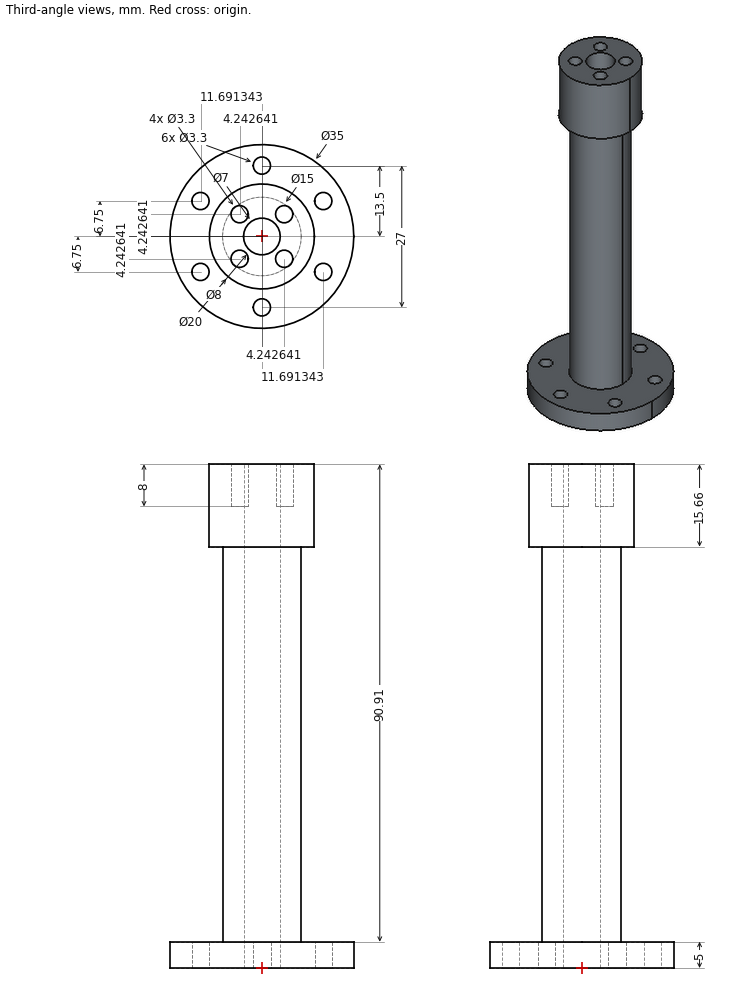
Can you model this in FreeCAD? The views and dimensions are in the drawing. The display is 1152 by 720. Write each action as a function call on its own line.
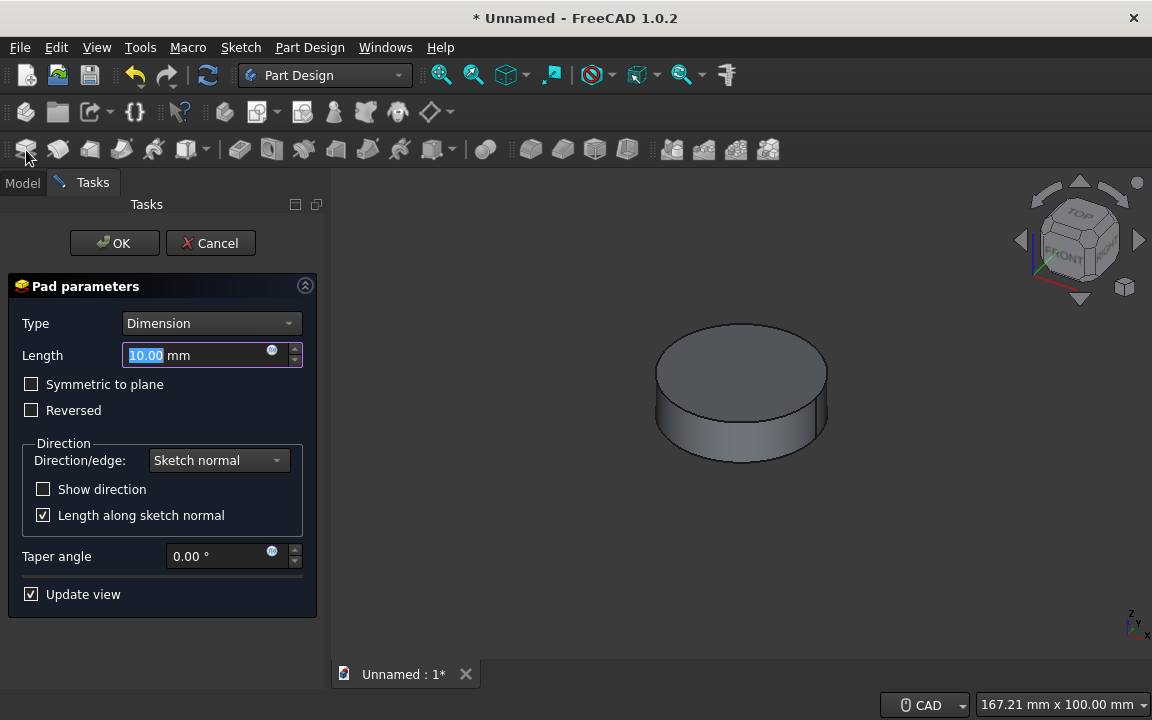
text(5)
key(Tab)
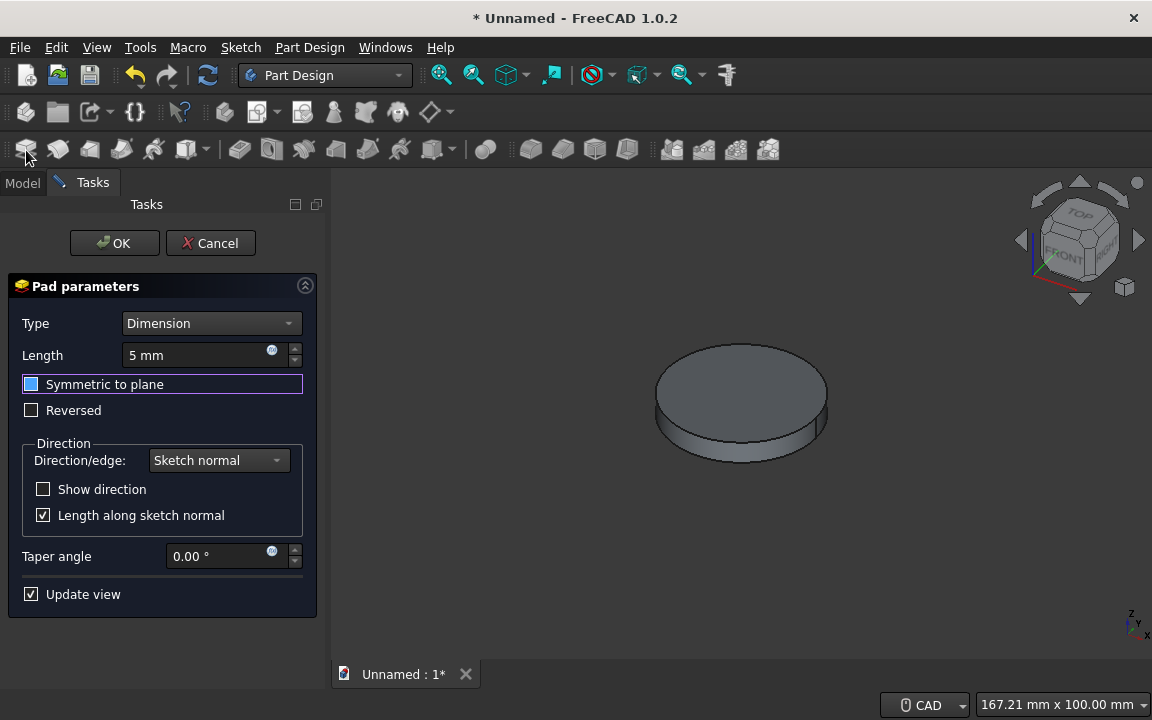
click(115, 243)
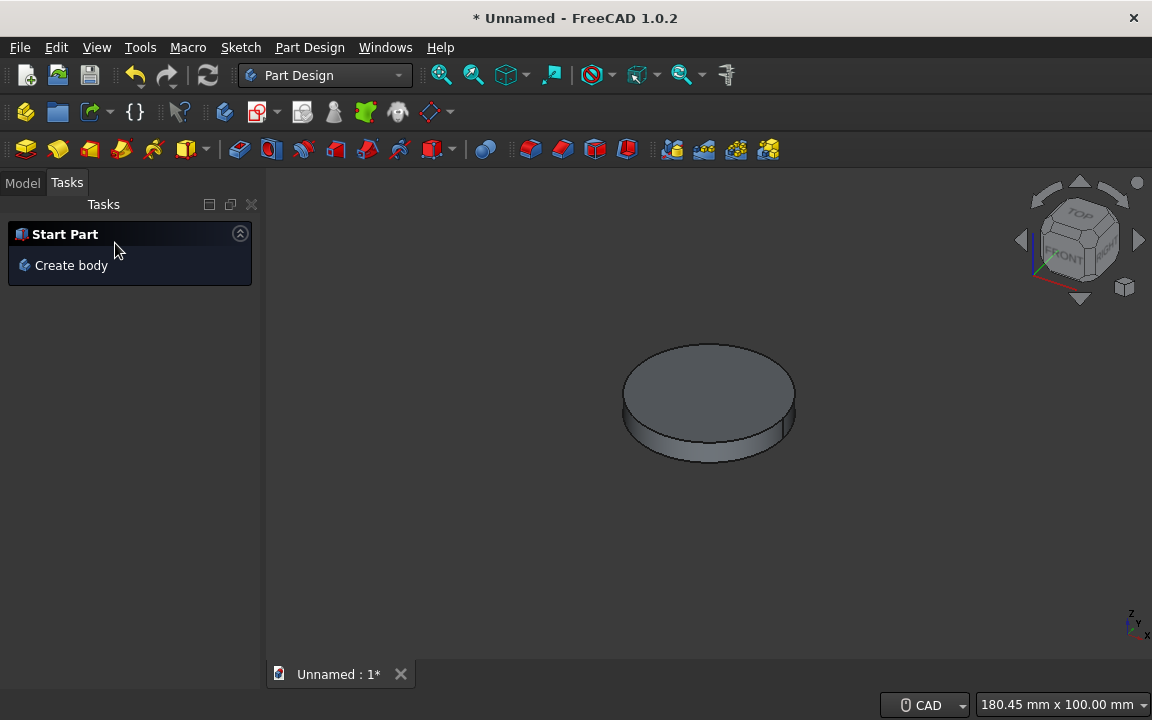
key(v)
key(f)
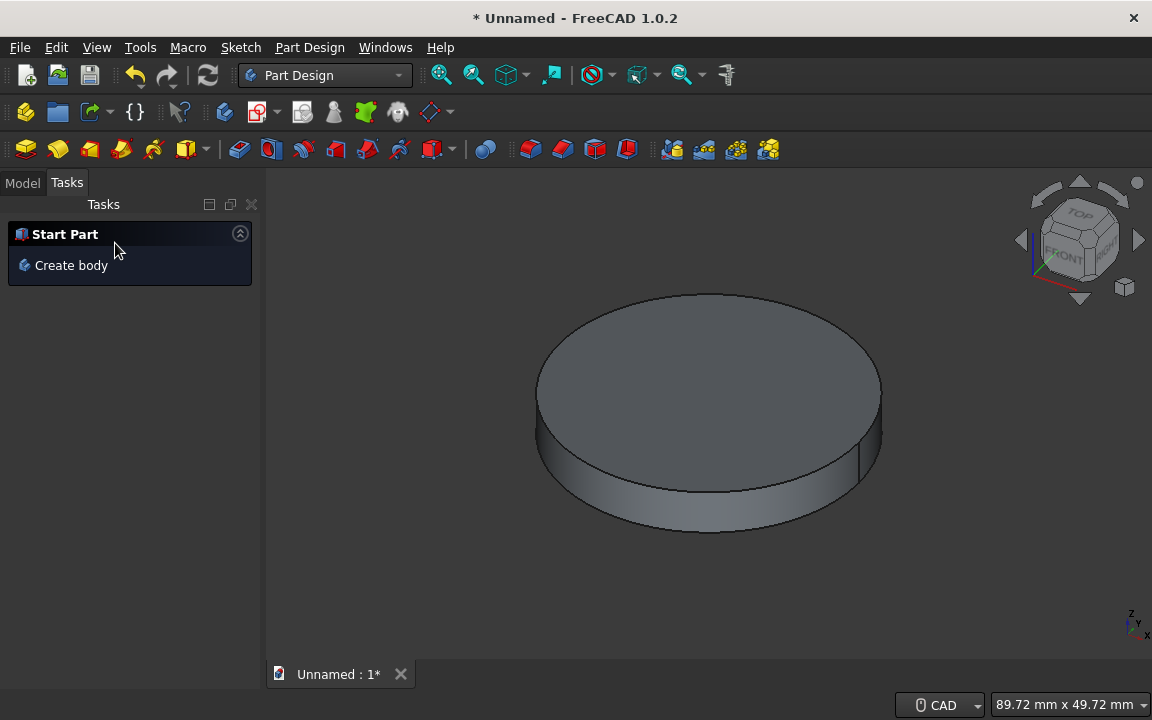
click(709, 392)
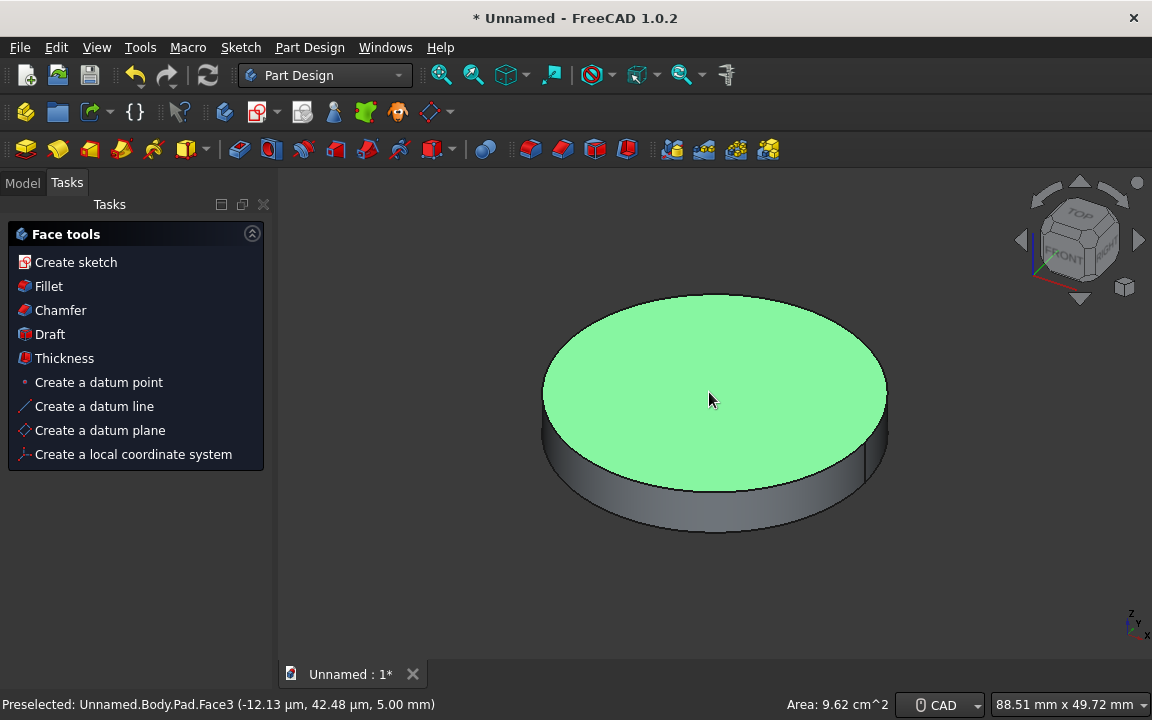
click(258, 112)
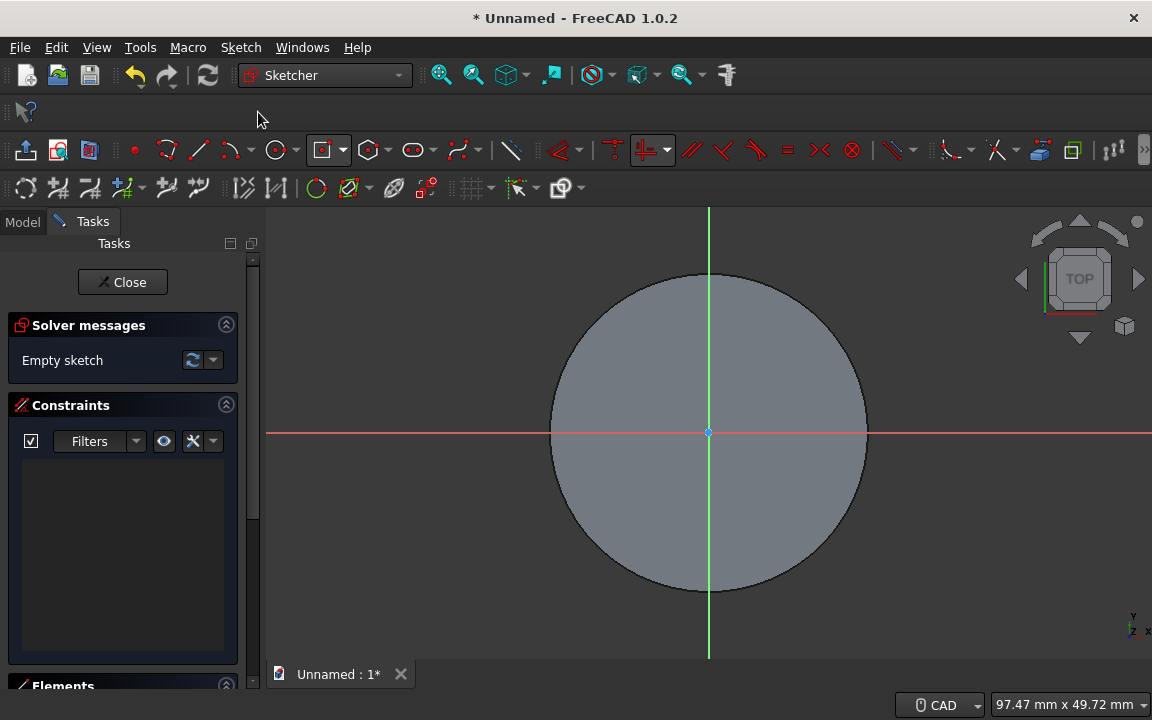
scroll(765, 433, up, 4)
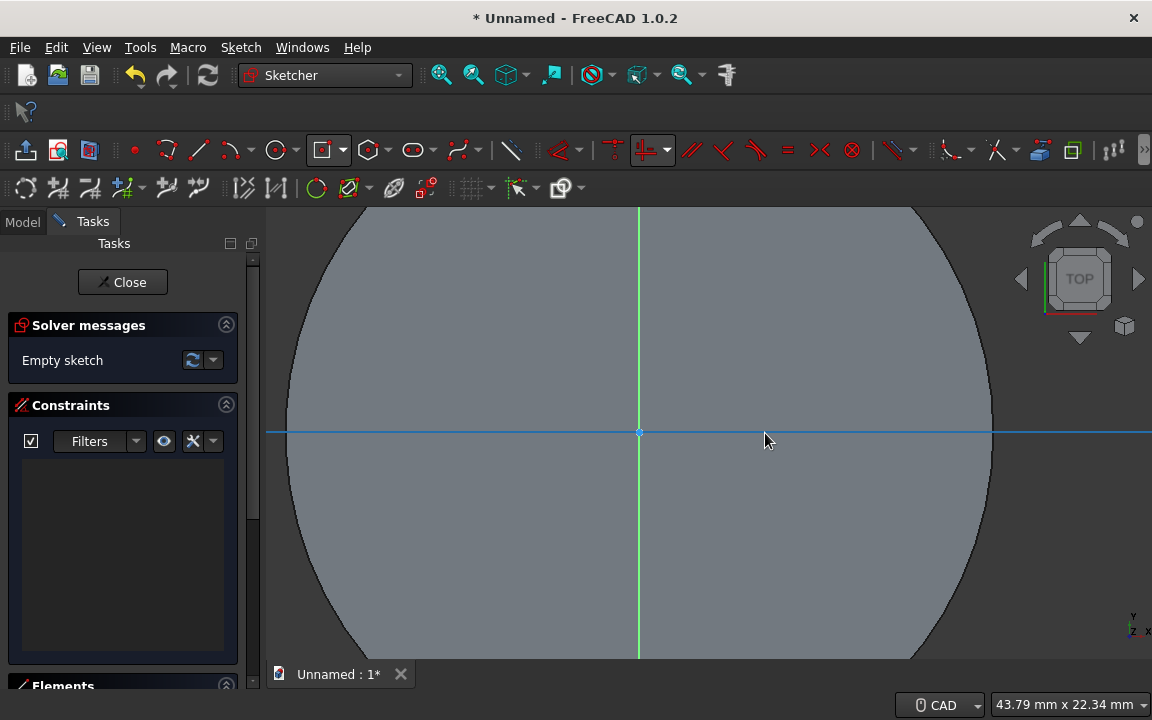
click(276, 150)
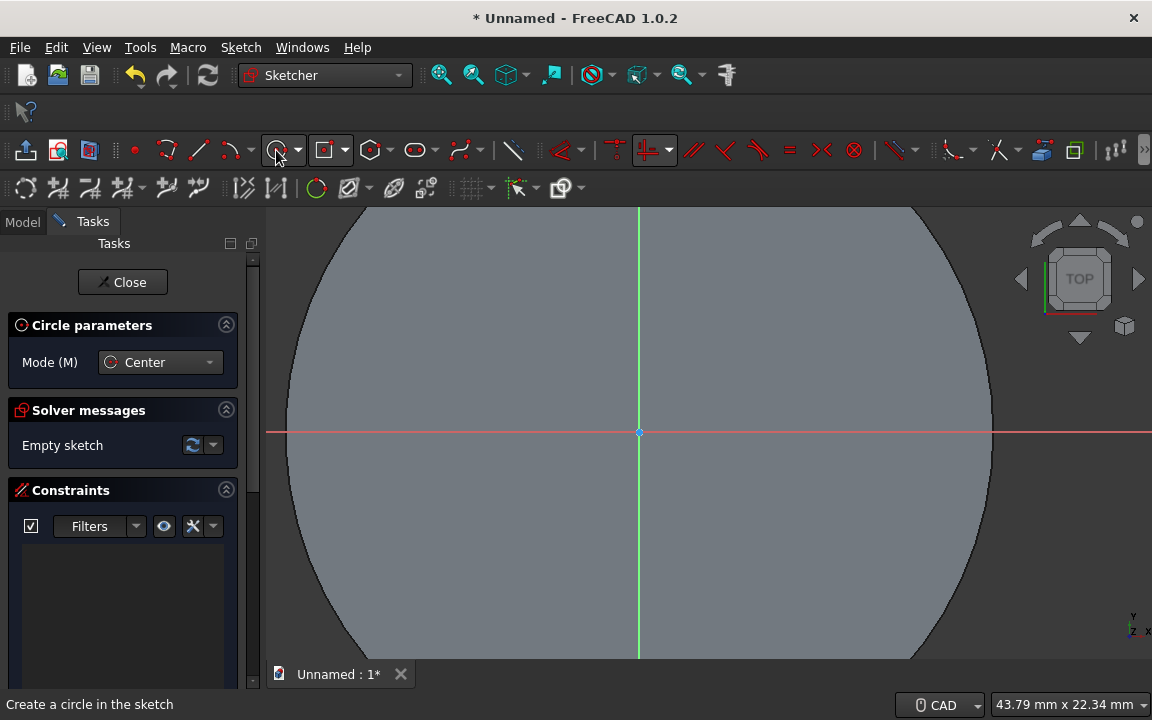
click(639, 432)
click(747, 325)
key(Escape)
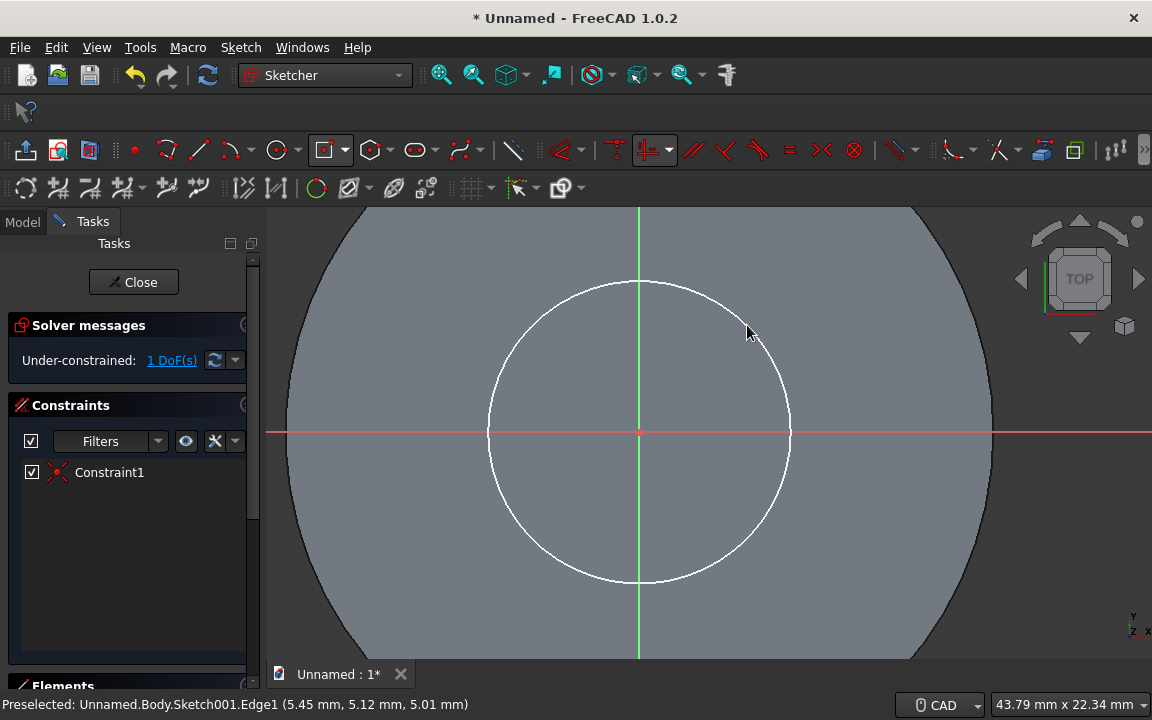
click(560, 150)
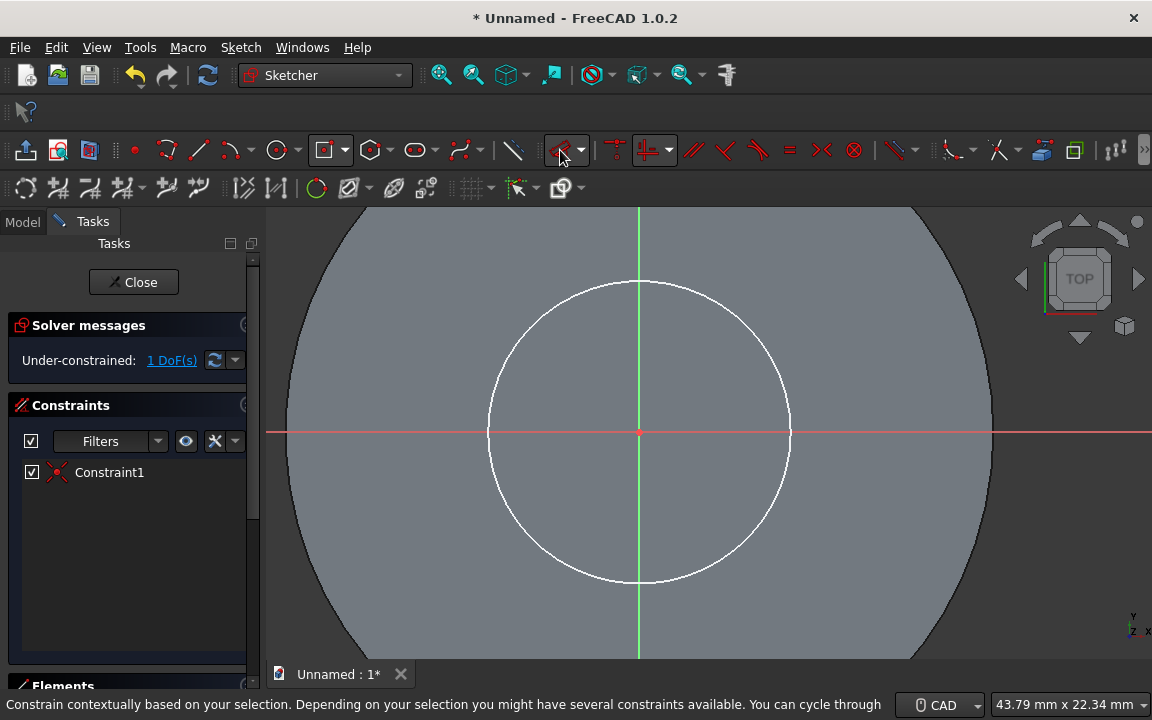
click(746, 325)
click(769, 302)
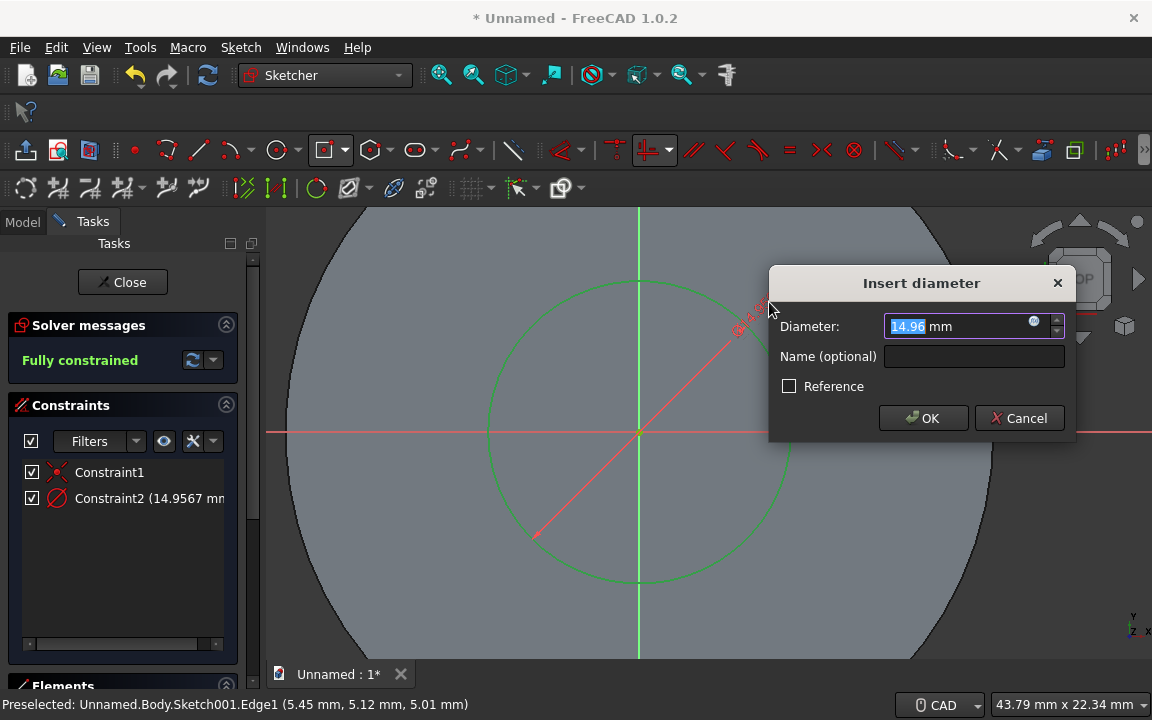
text(15)
key(Return)
key(Escape)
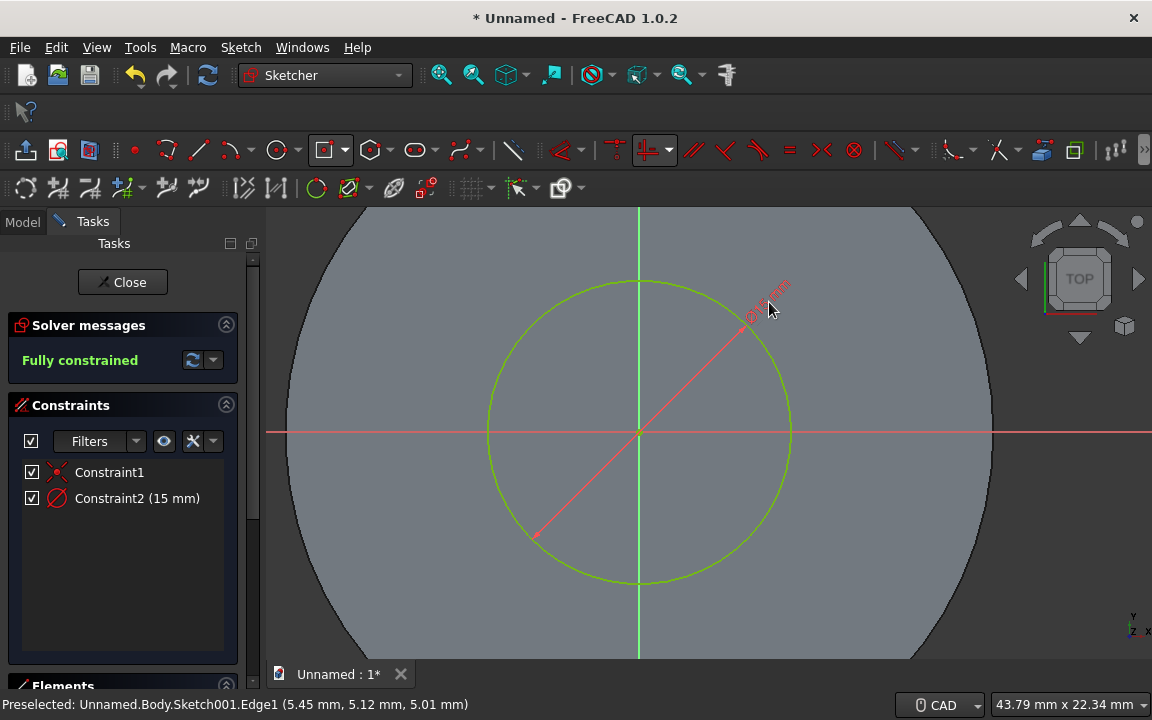
click(123, 282)